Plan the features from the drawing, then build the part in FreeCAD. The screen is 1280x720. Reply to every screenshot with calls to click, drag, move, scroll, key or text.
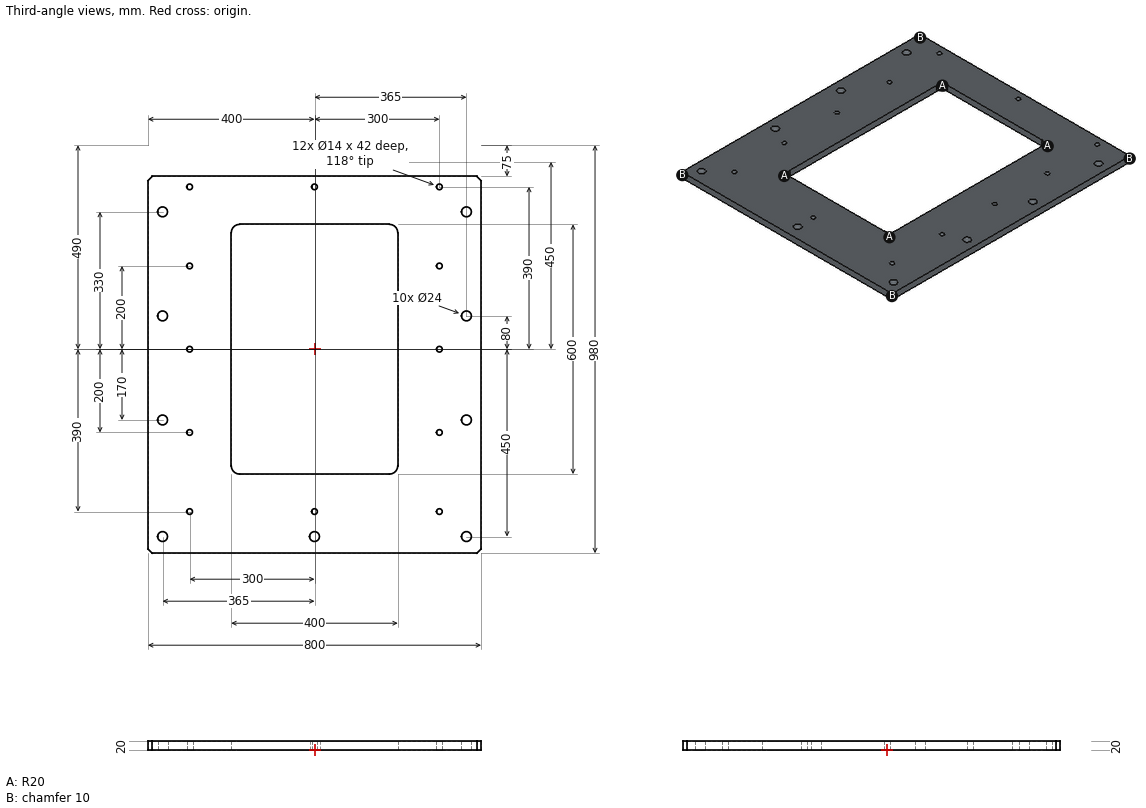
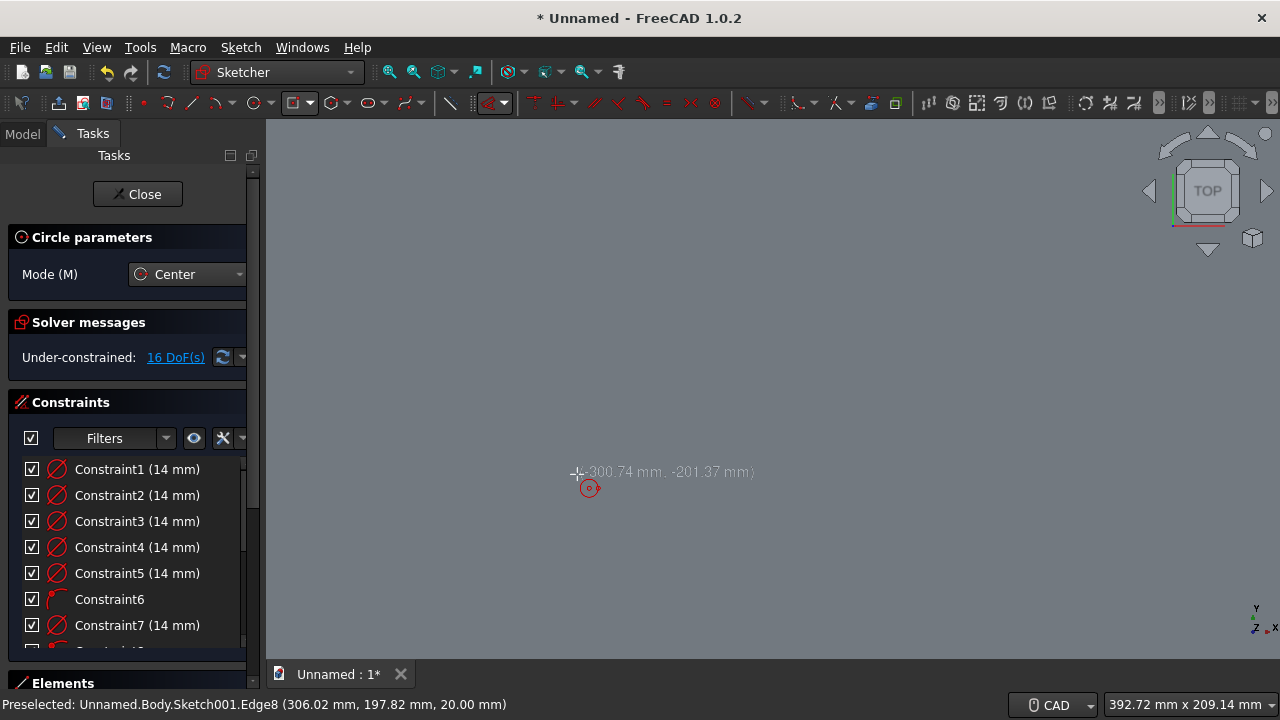
scroll(576, 475, down, 11)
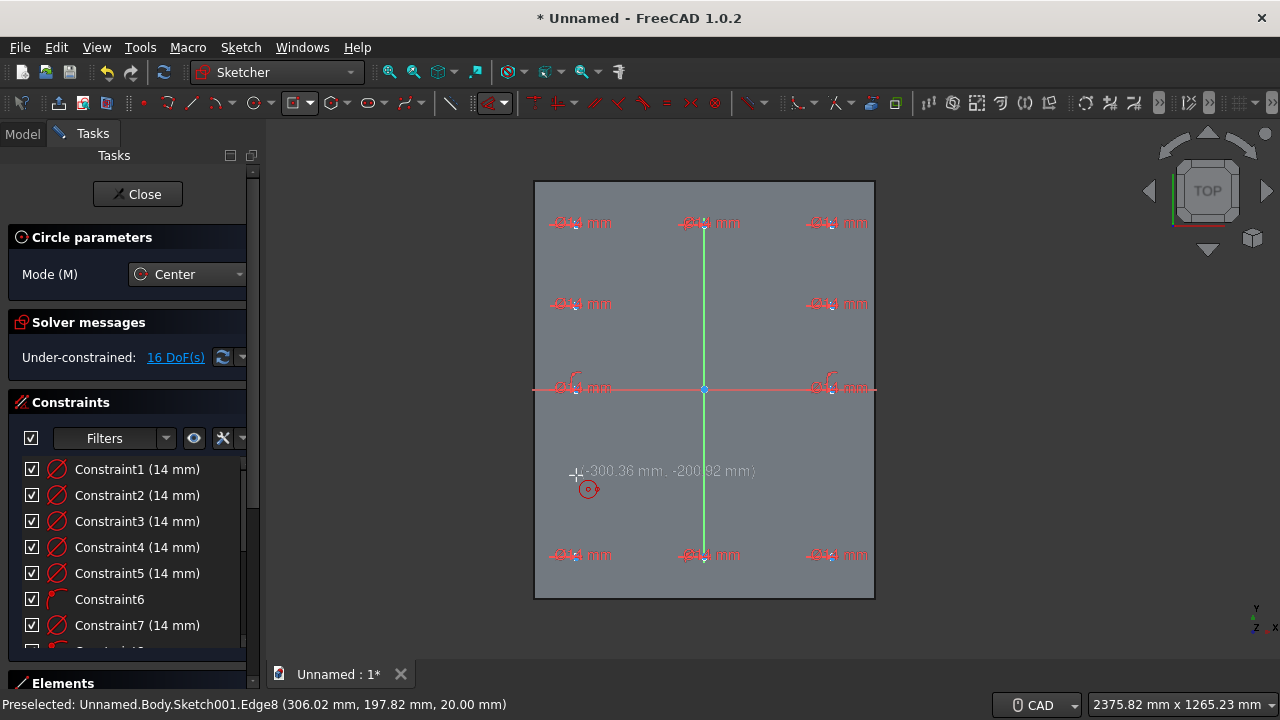
click(576, 475)
move(579, 473)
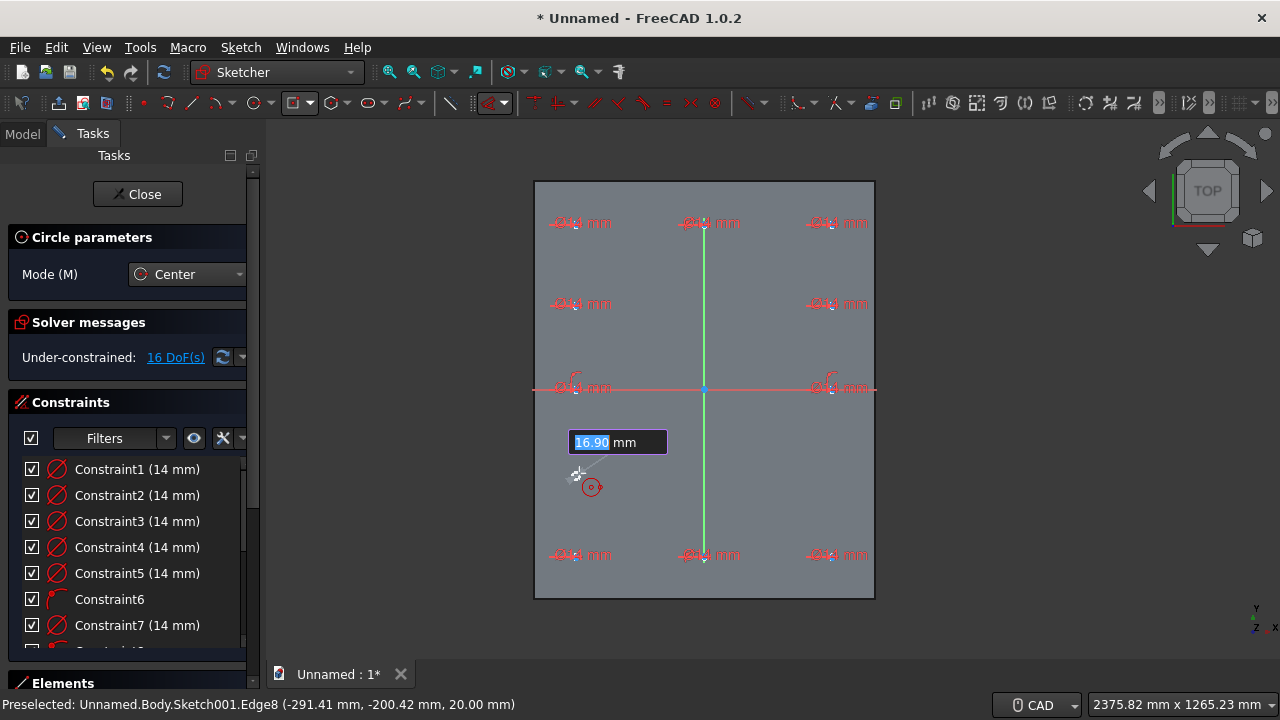
text(14)
key(Return)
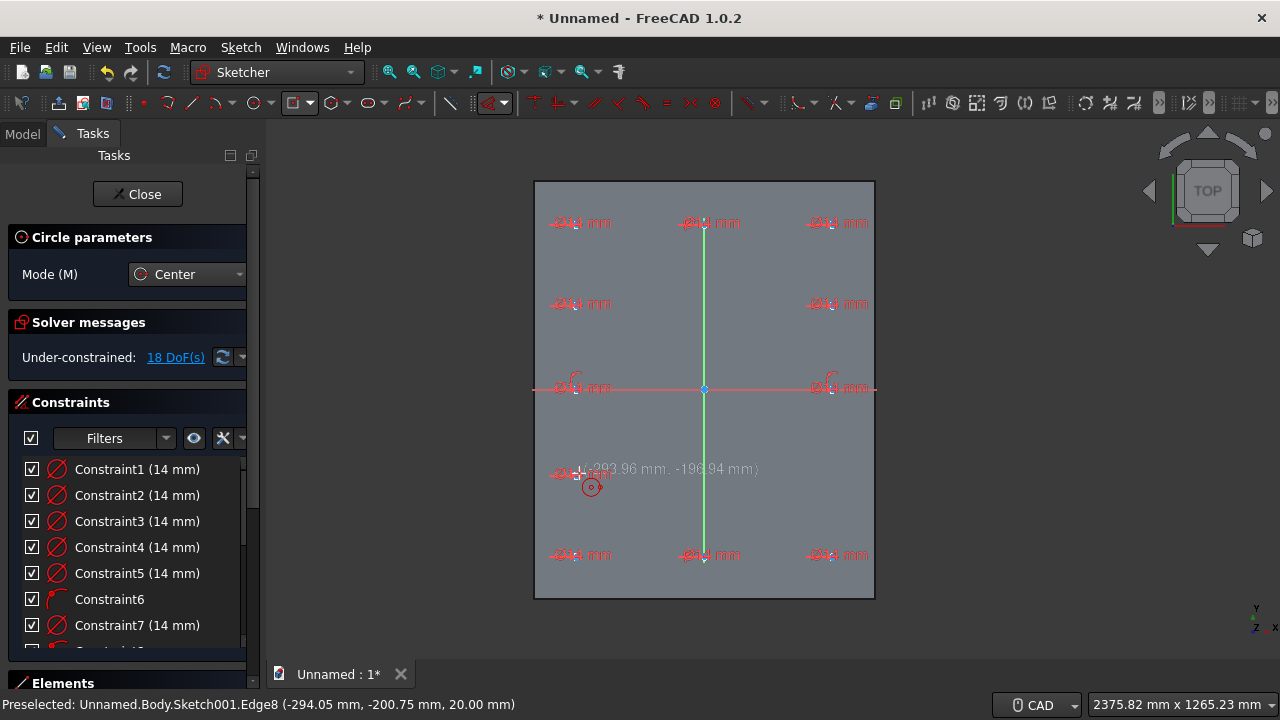
scroll(833, 475, up, 11)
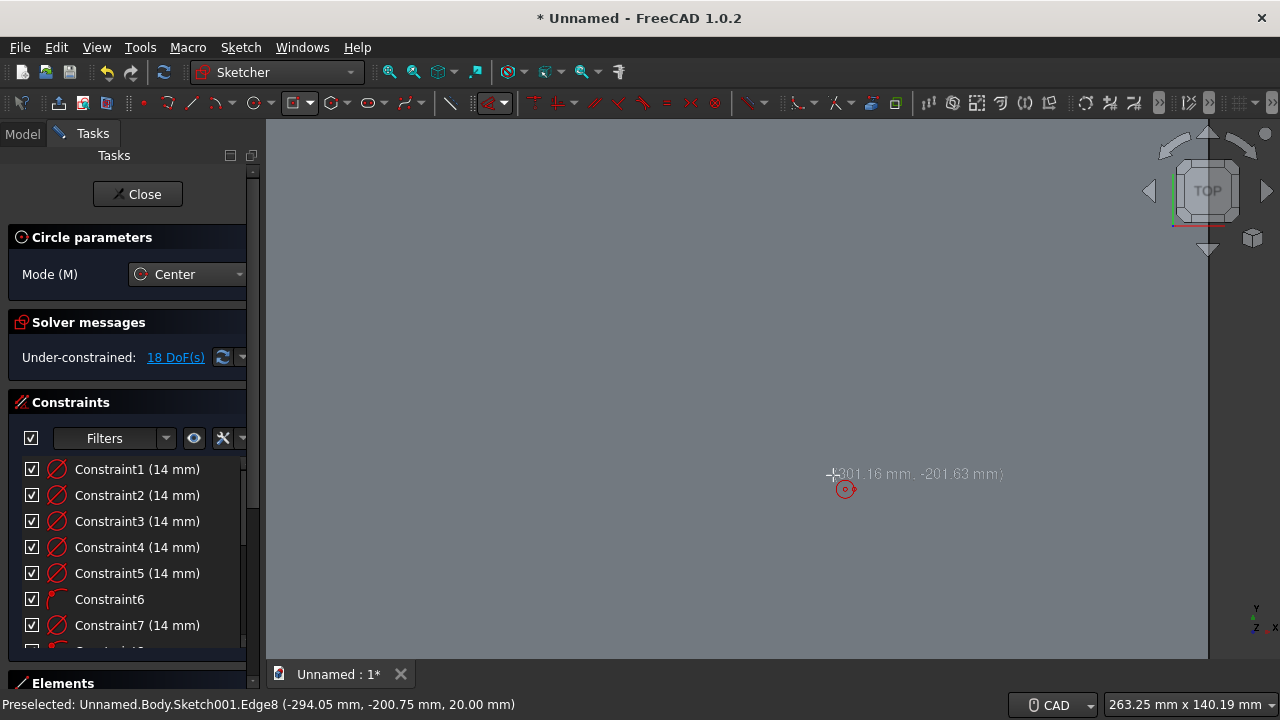
scroll(834, 475, down, 11)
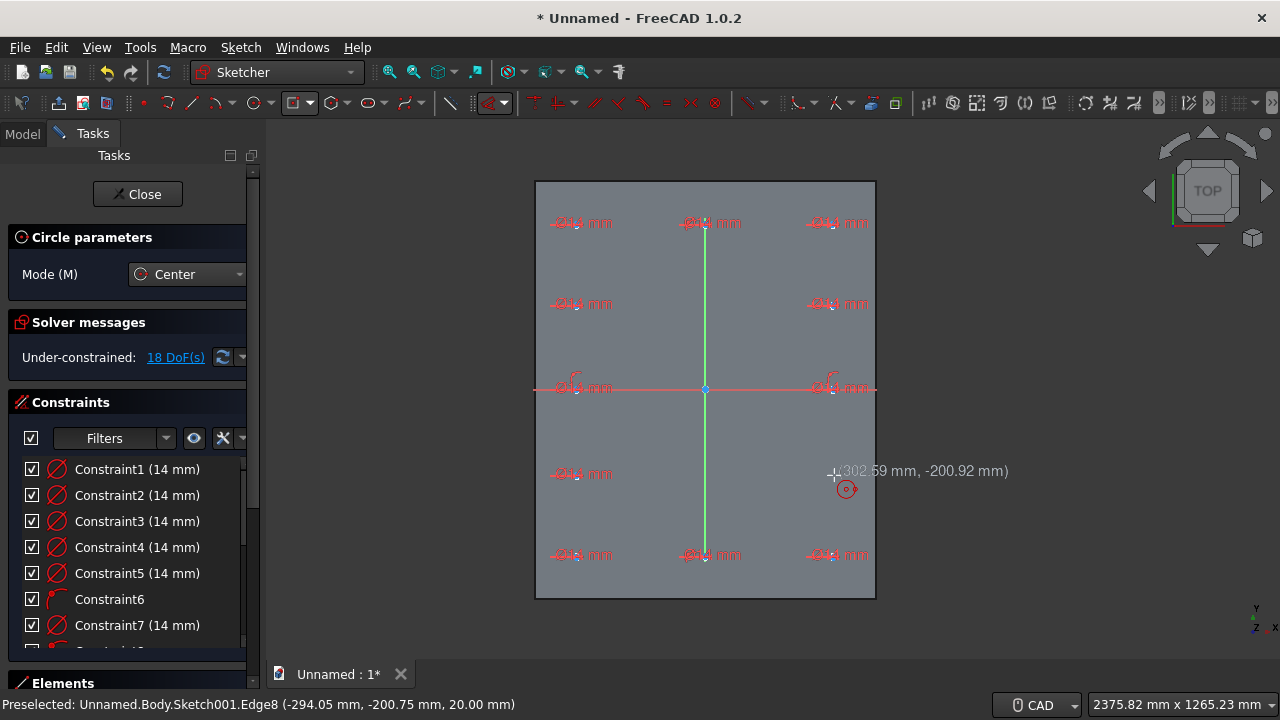
click(833, 475)
move(836, 473)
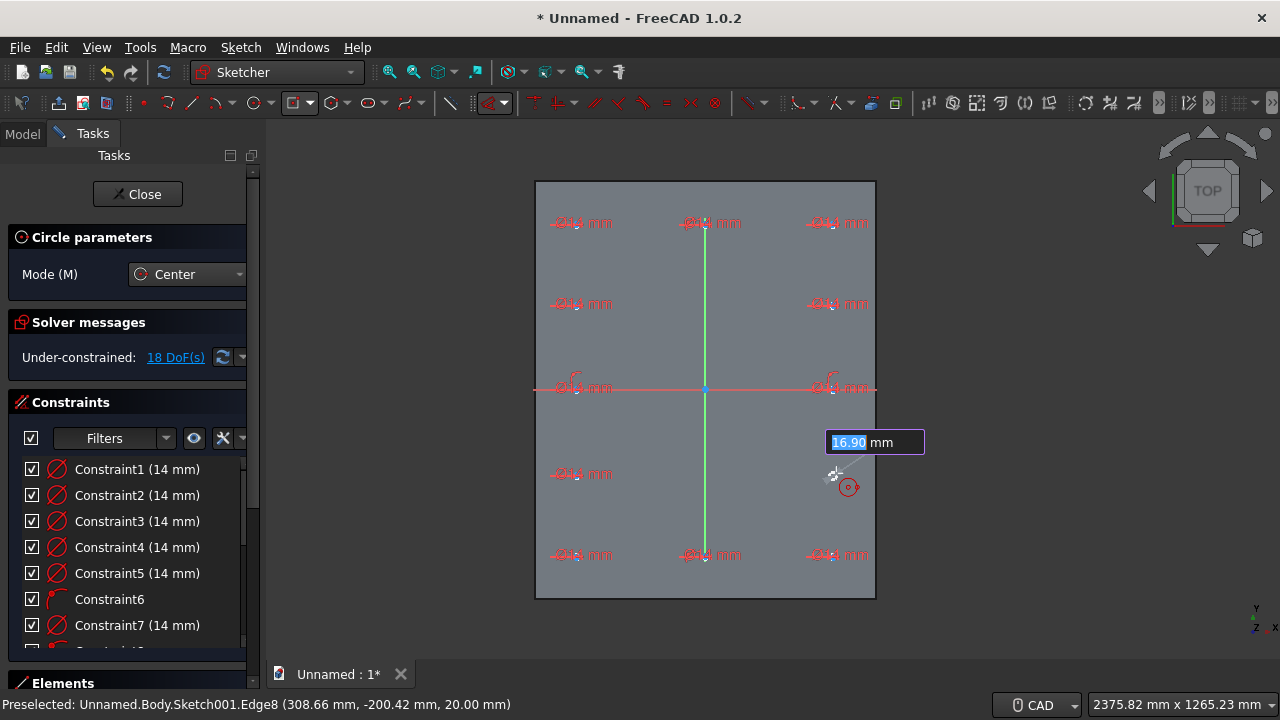
text(14)
key(Return)
key(Escape)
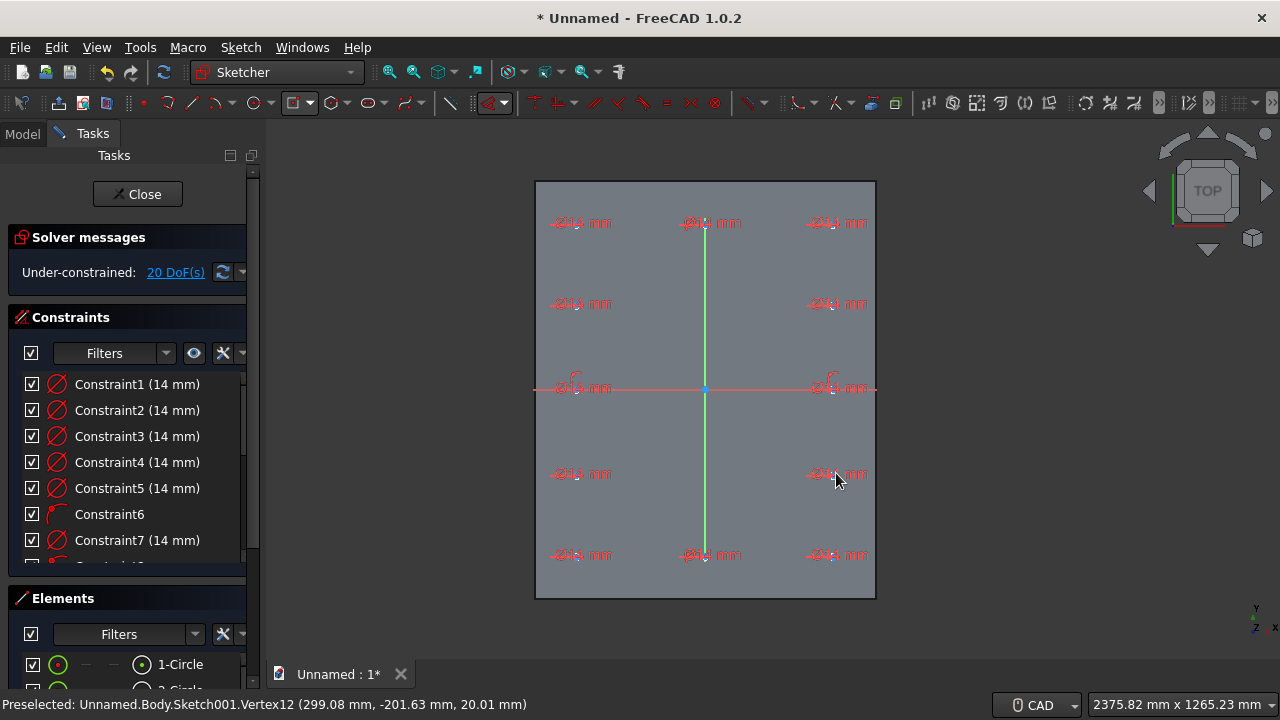
click(577, 557)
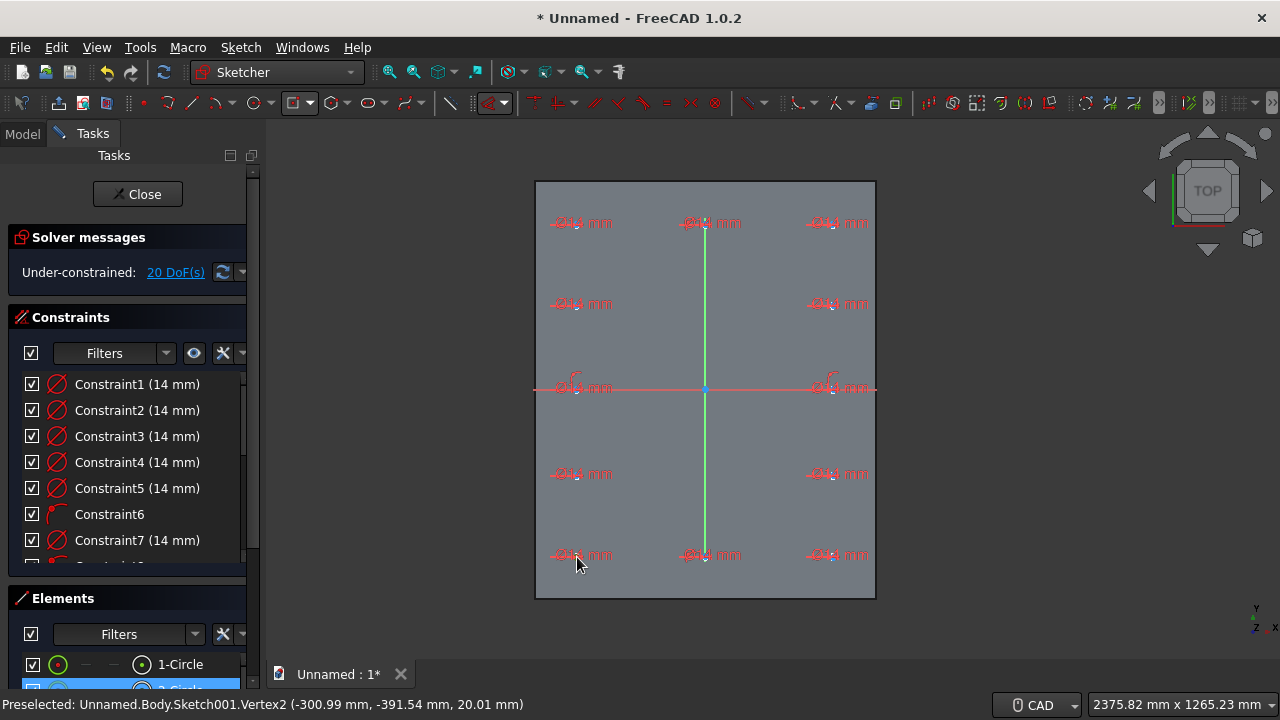
click(577, 225)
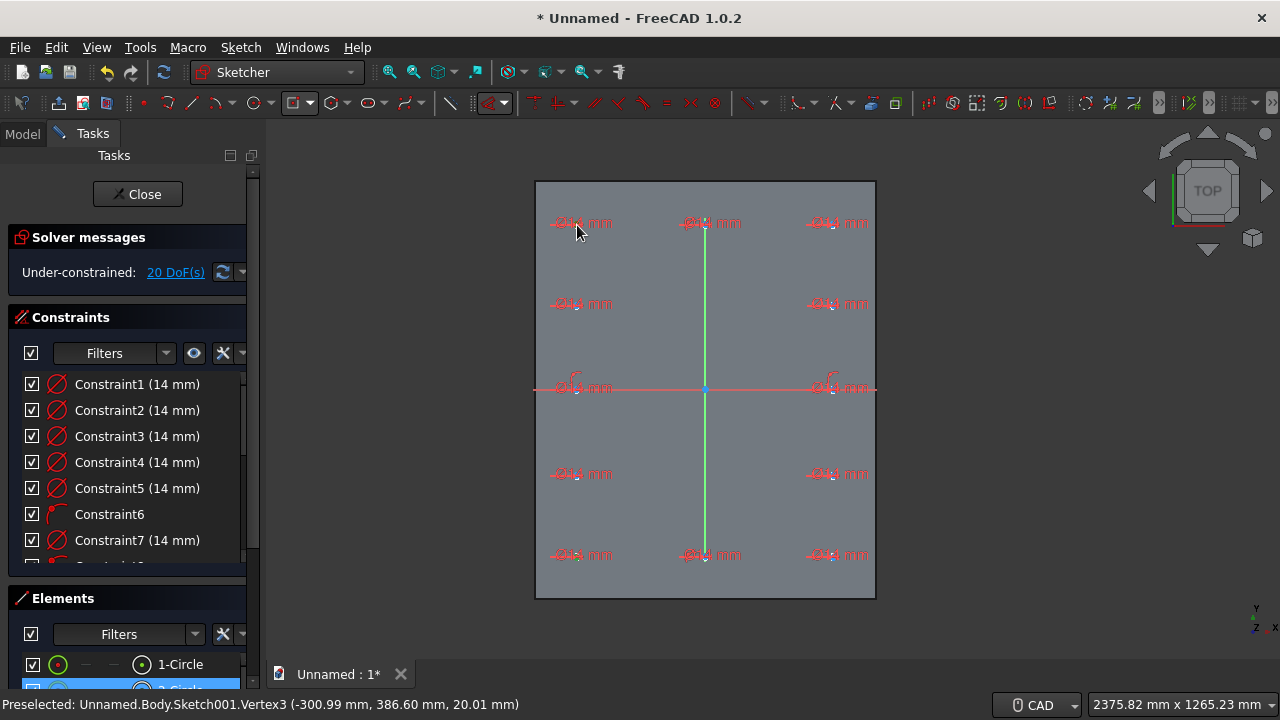
click(576, 104)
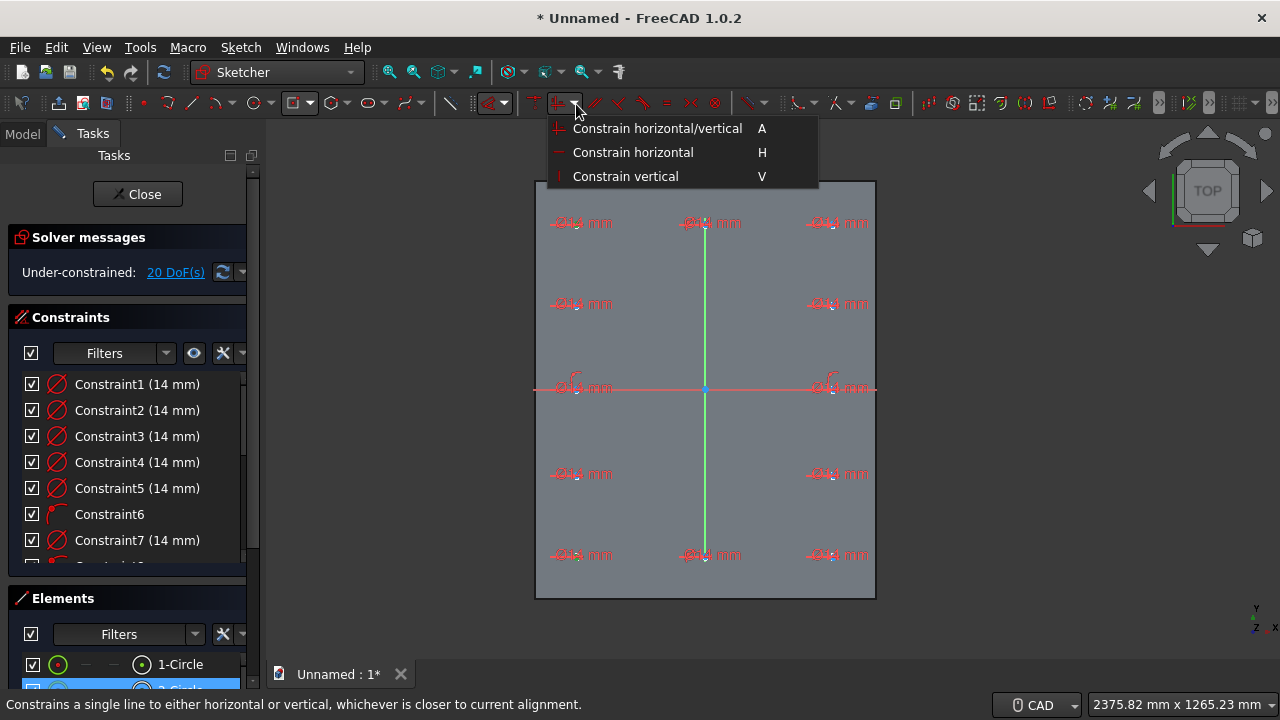
click(683, 176)